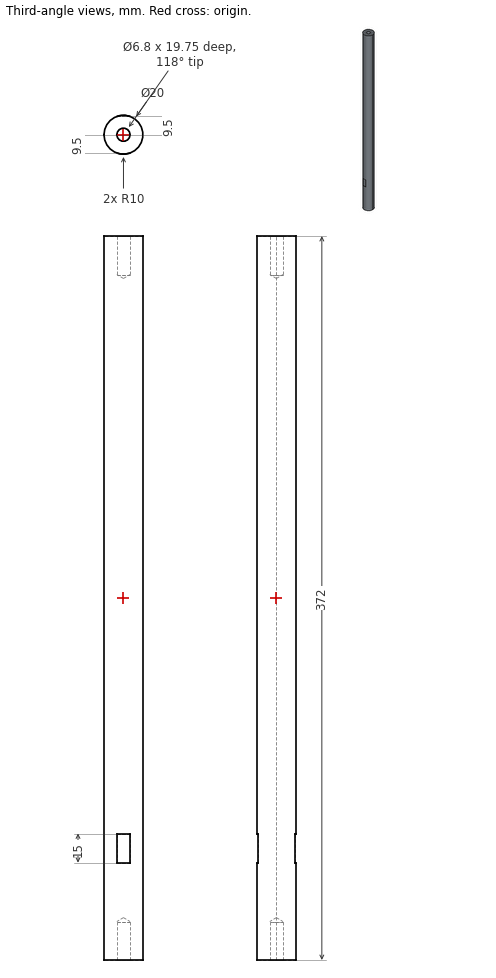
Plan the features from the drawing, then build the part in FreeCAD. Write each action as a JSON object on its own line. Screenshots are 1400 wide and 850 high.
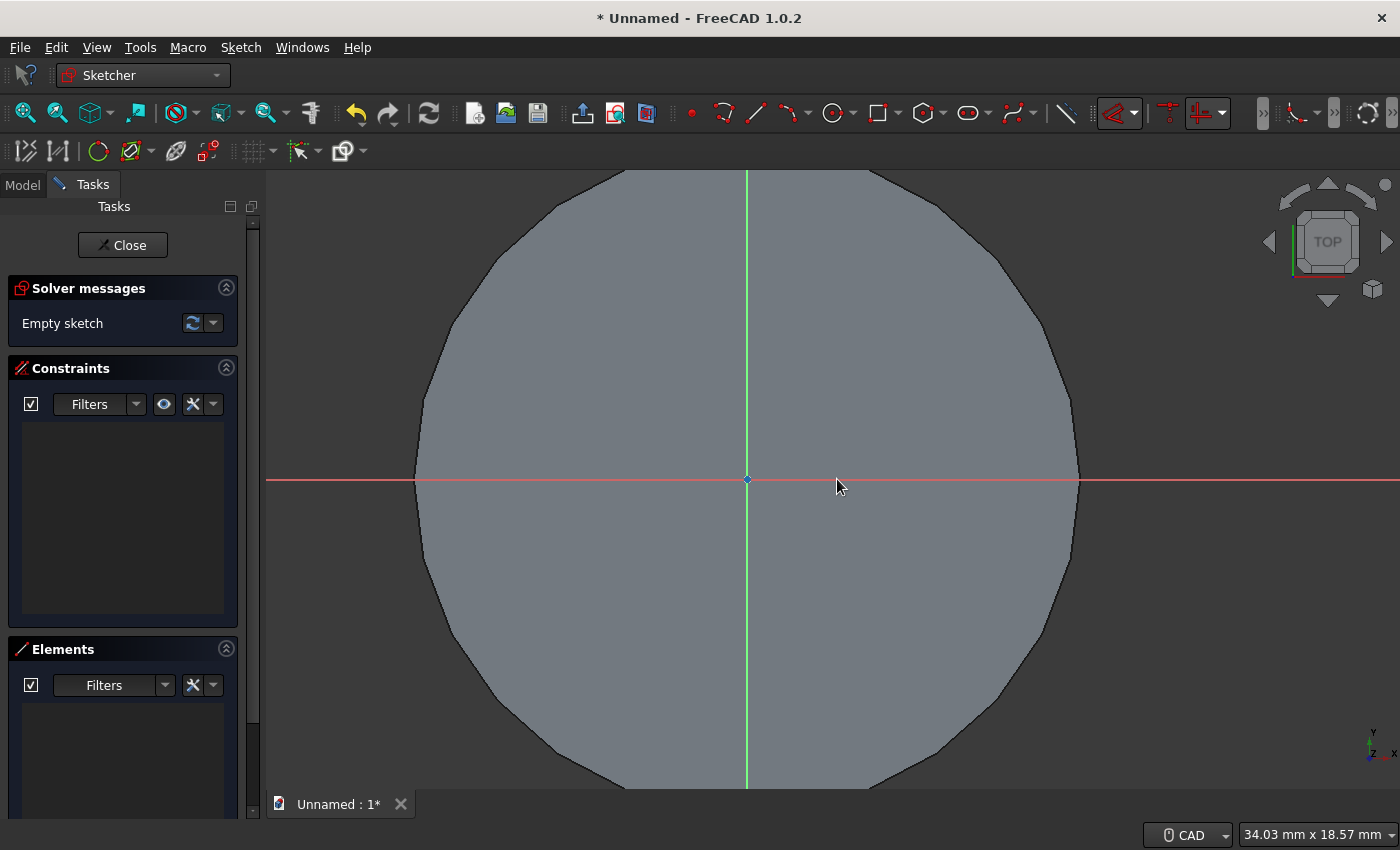
{"action": "scroll", "coordinate": [726, 480], "scroll_direction": "up", "scroll_amount": 3}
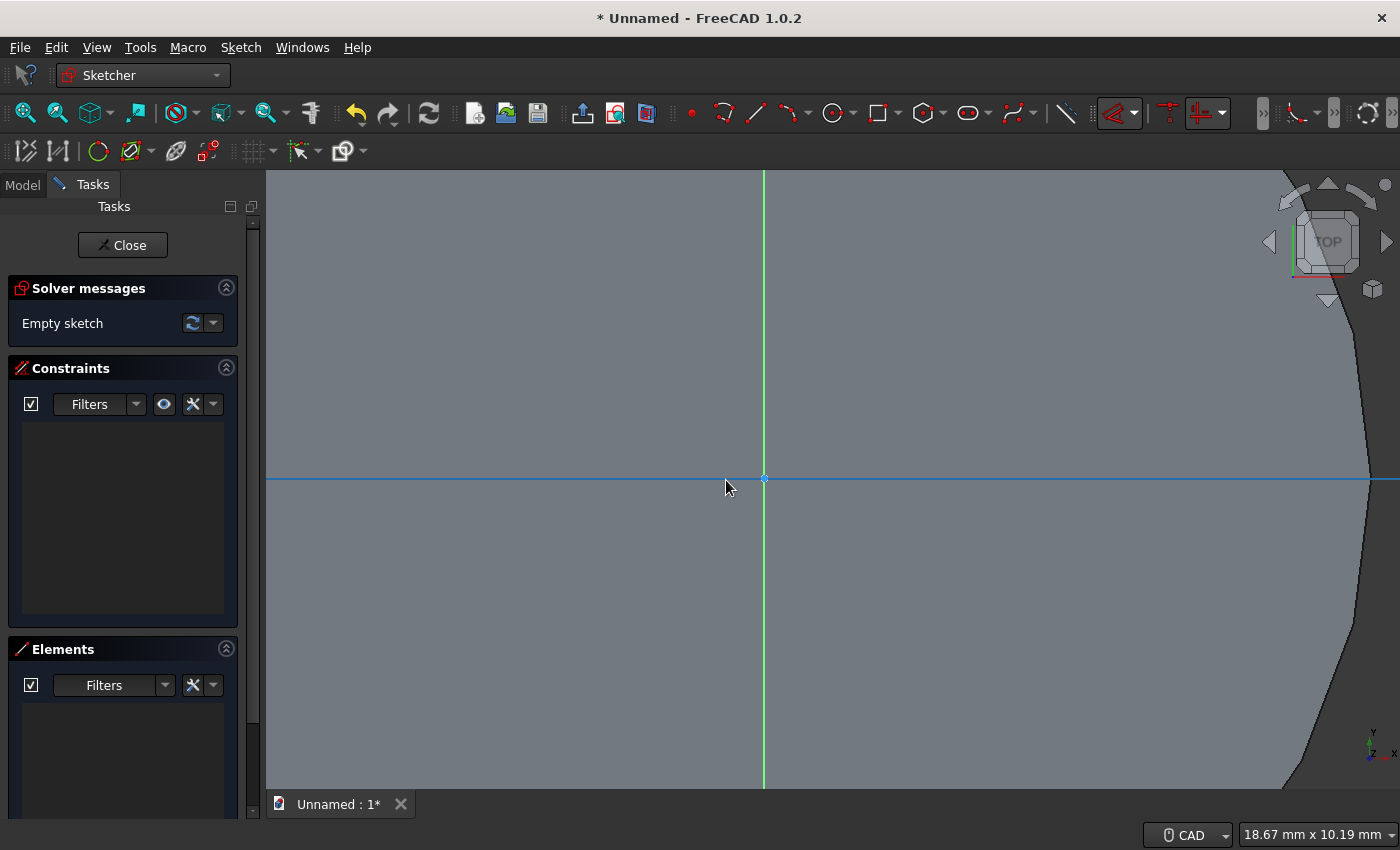
{"action": "left_click", "coordinate": [834, 114]}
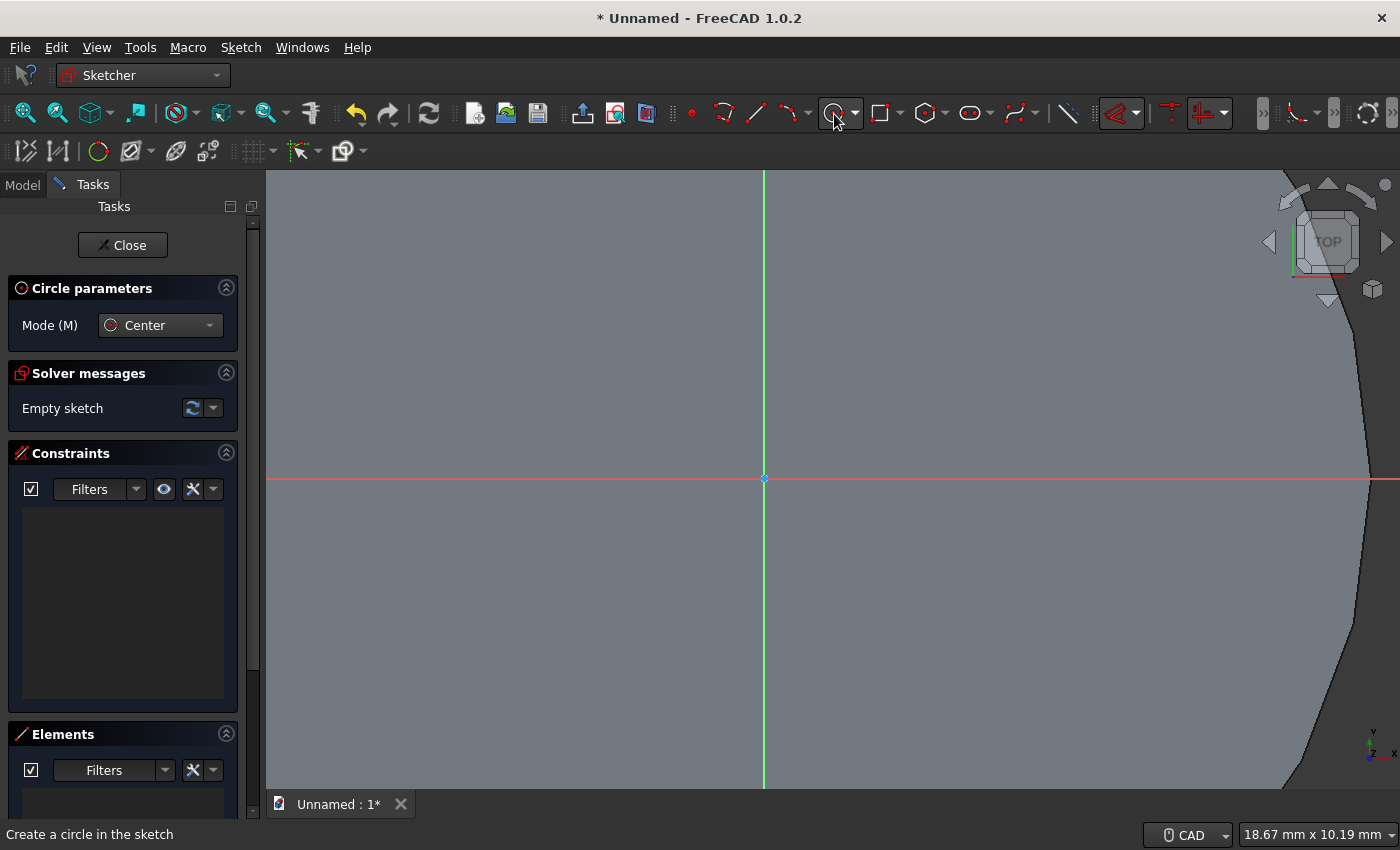
{"action": "left_click", "coordinate": [764, 479]}
{"action": "left_click", "coordinate": [910, 333]}
{"action": "key", "text": "Escape"}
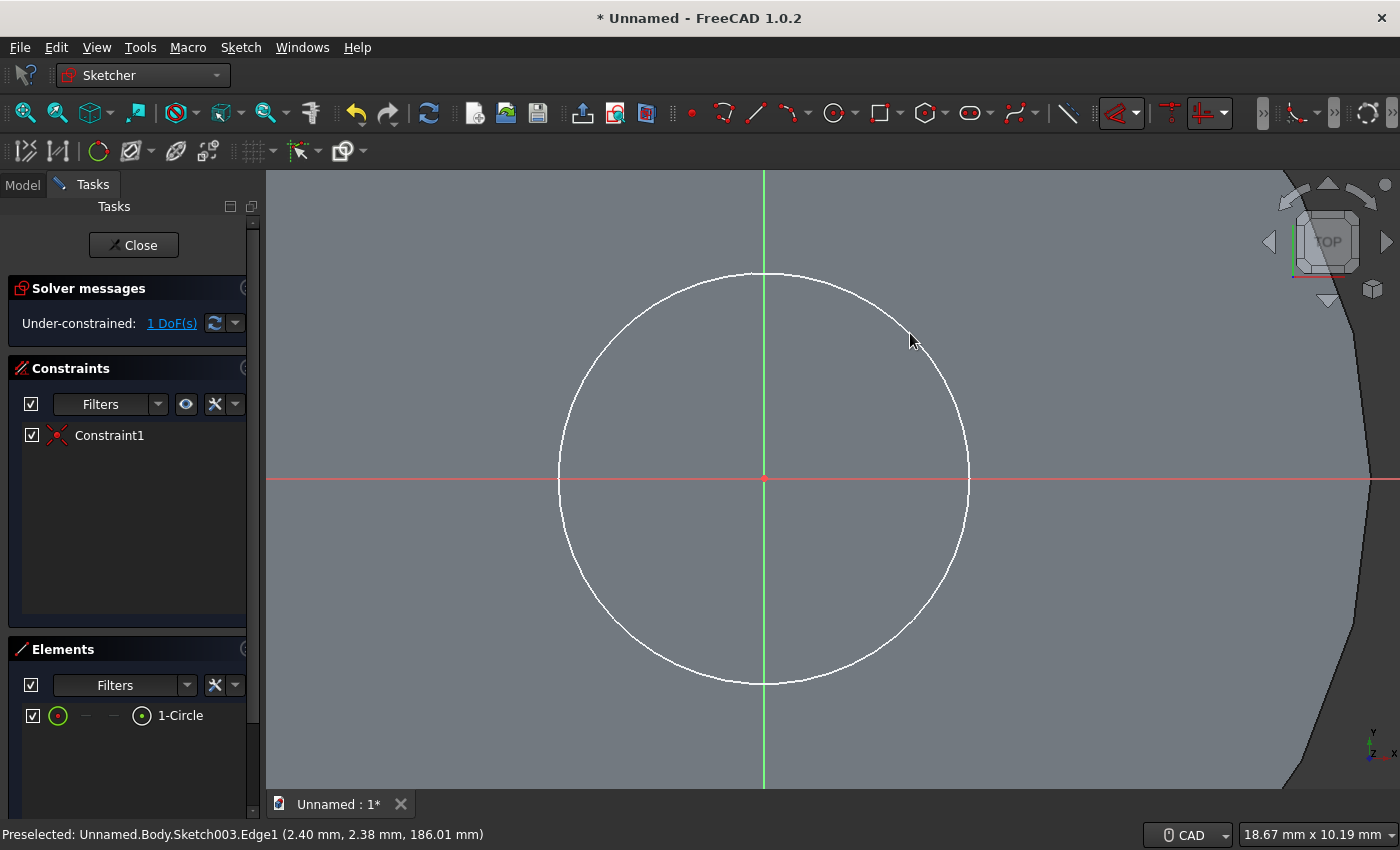
{"action": "left_click", "coordinate": [909, 333]}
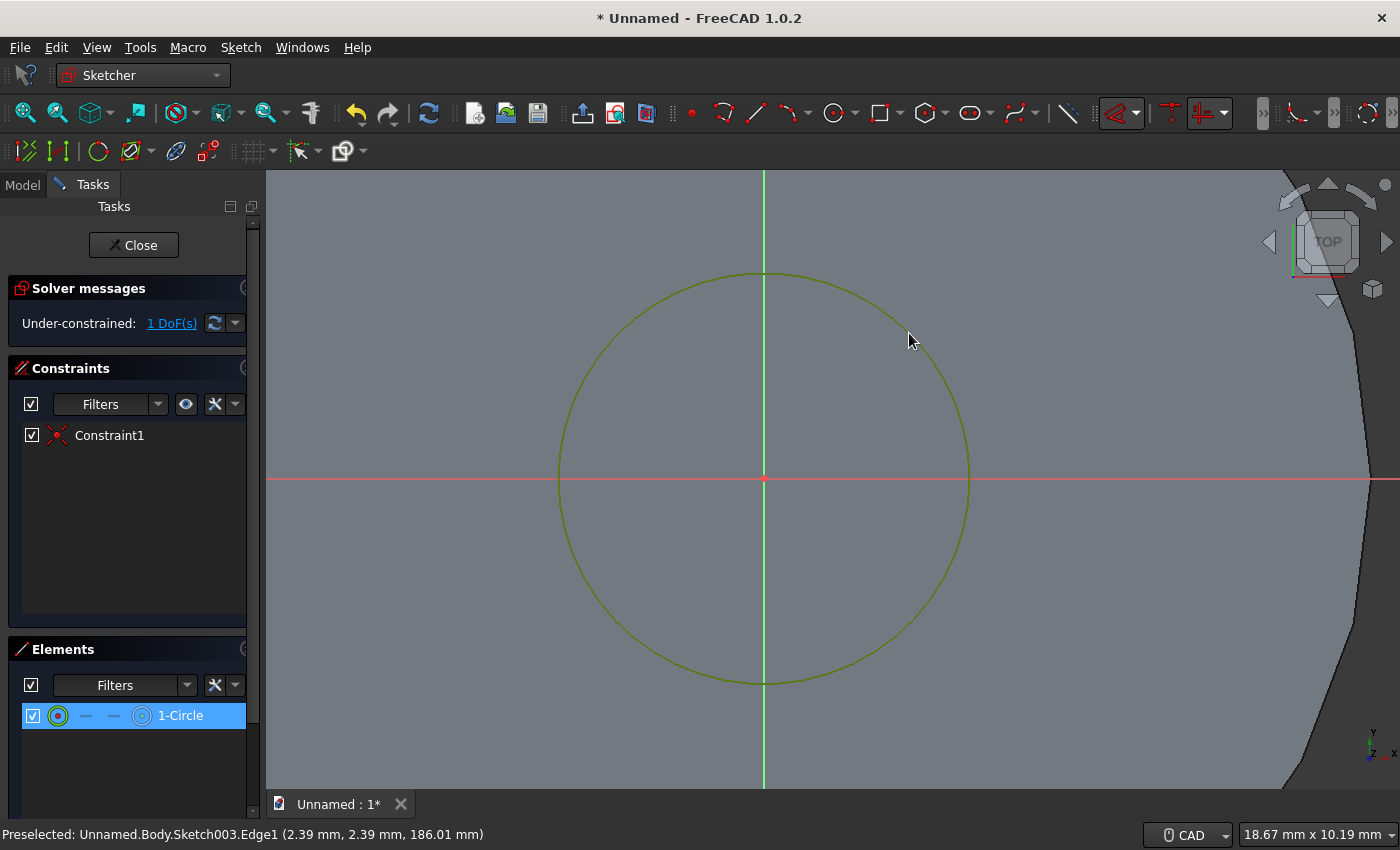
{"action": "key", "text": "k o"}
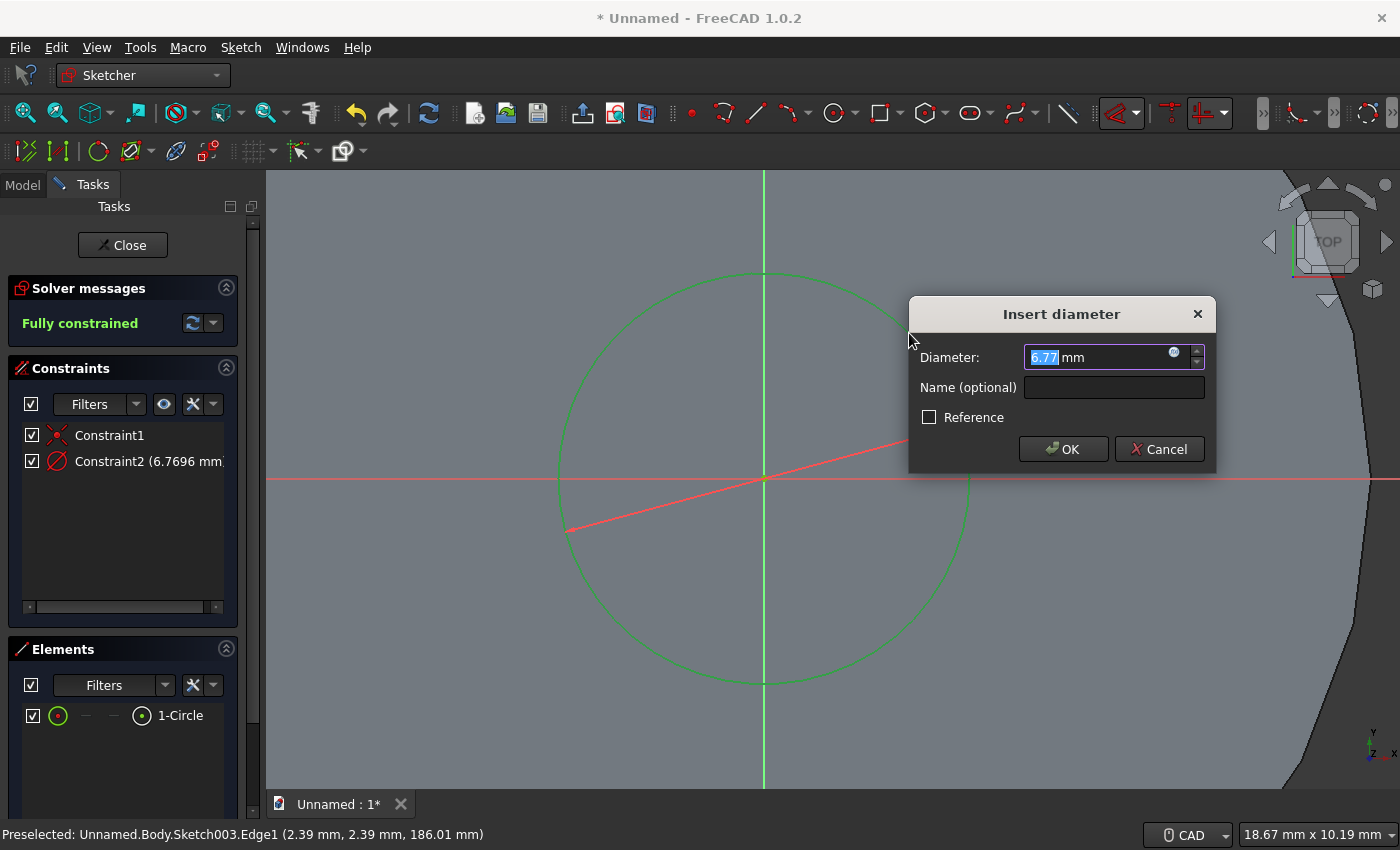
{"action": "type", "text": "6.8"}
{"action": "key", "text": "Return"}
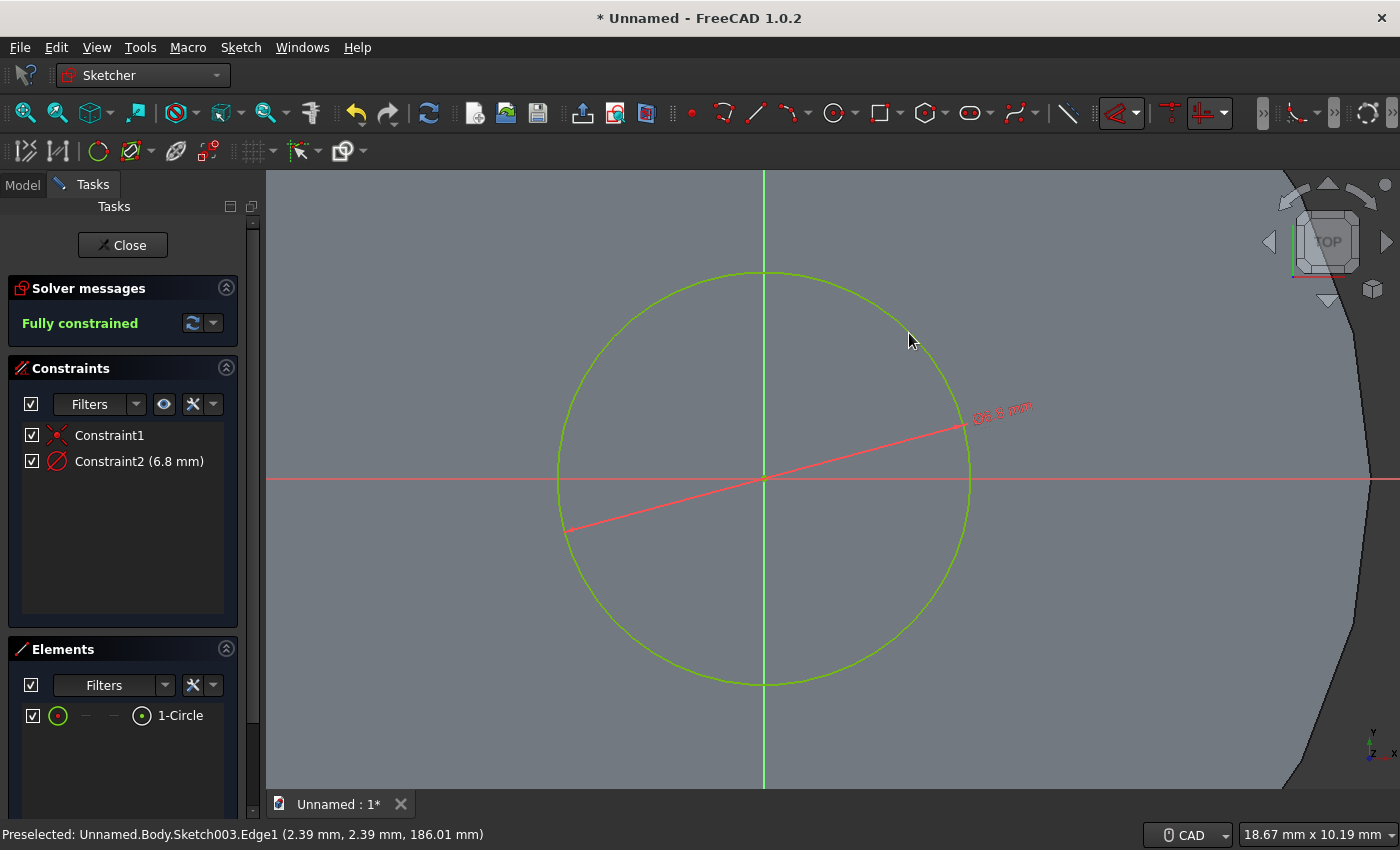
{"action": "left_click", "coordinate": [123, 245]}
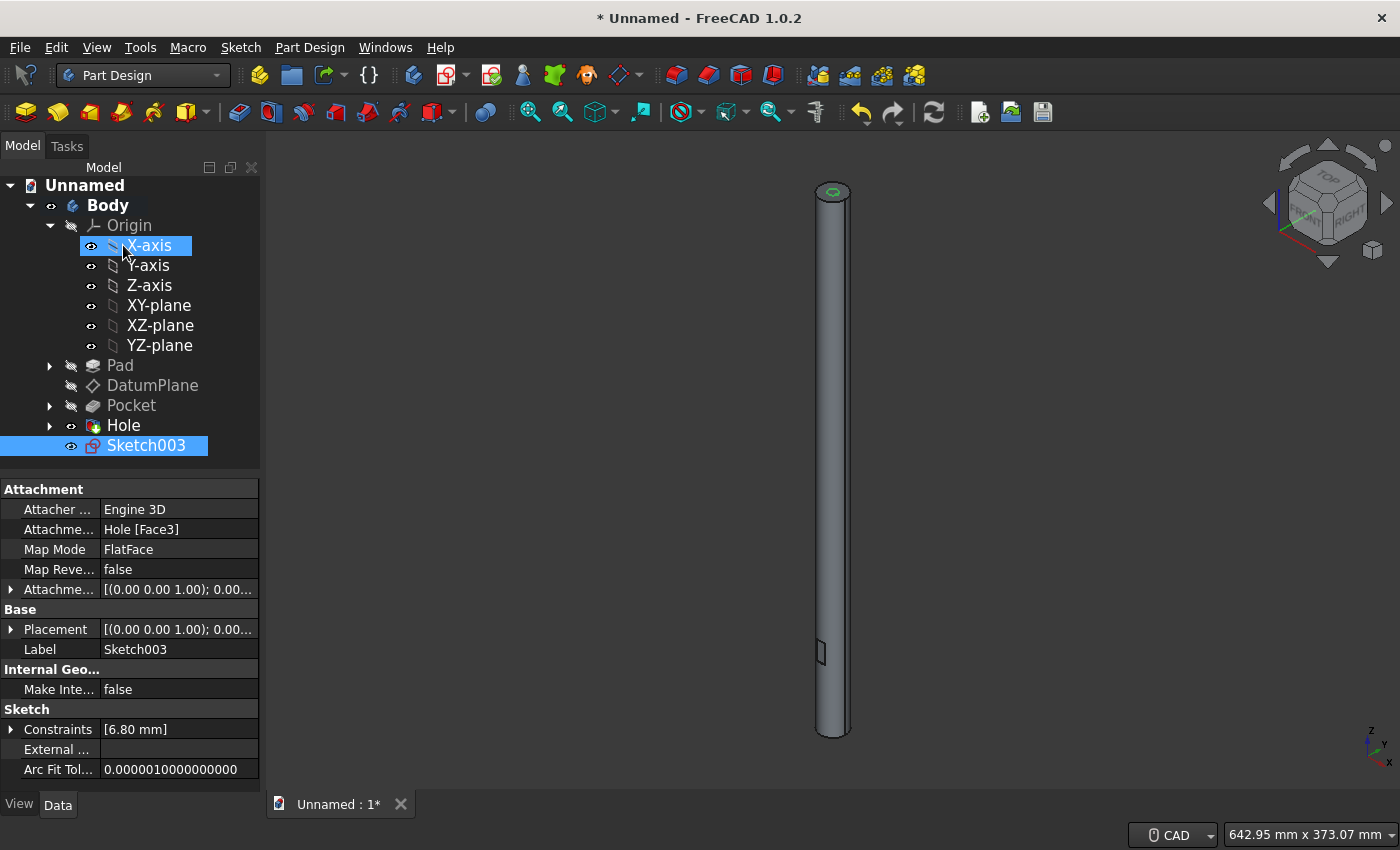
{"action": "left_click", "coordinate": [272, 112]}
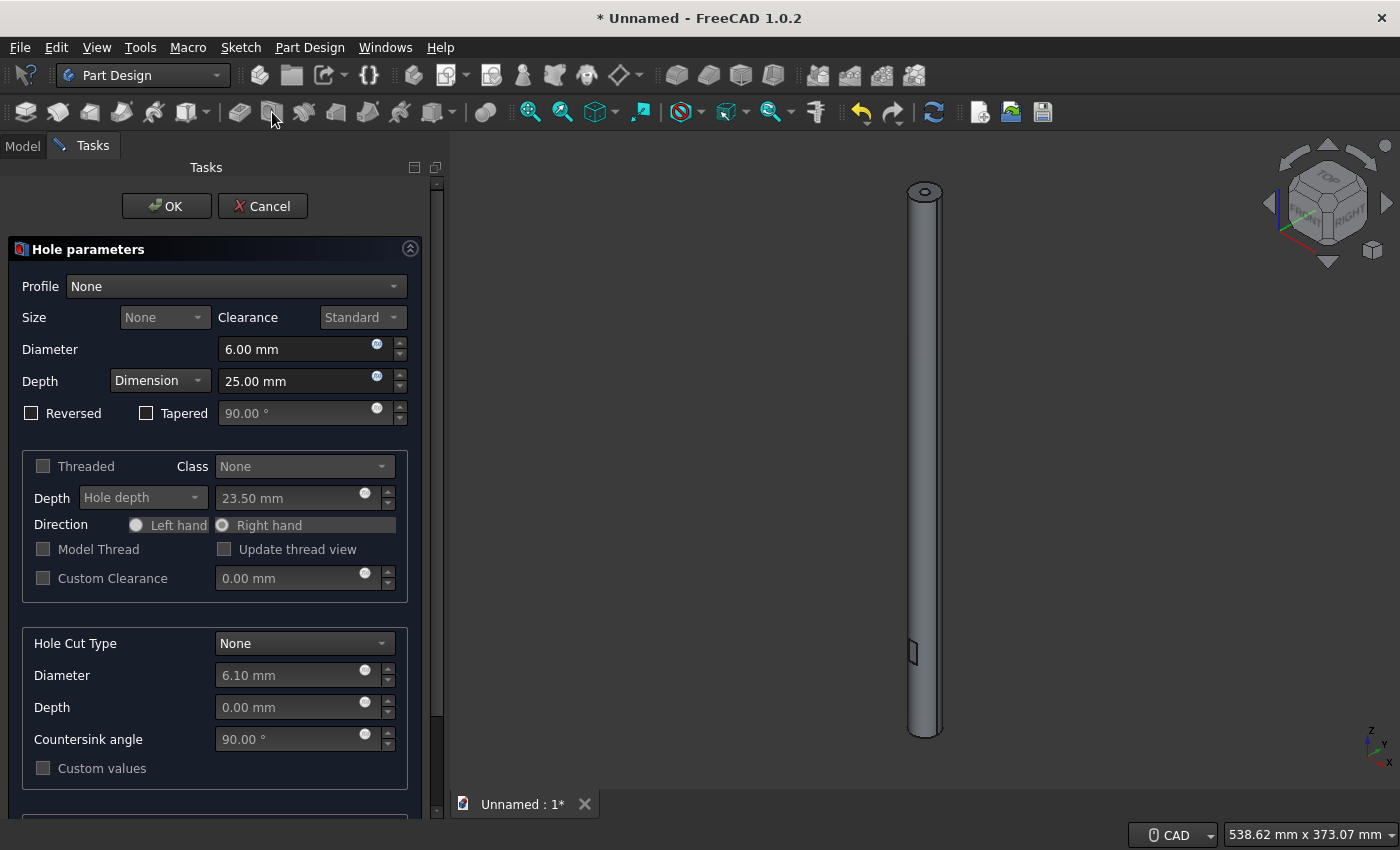
{"action": "triple_click", "coordinate": [305, 349]}